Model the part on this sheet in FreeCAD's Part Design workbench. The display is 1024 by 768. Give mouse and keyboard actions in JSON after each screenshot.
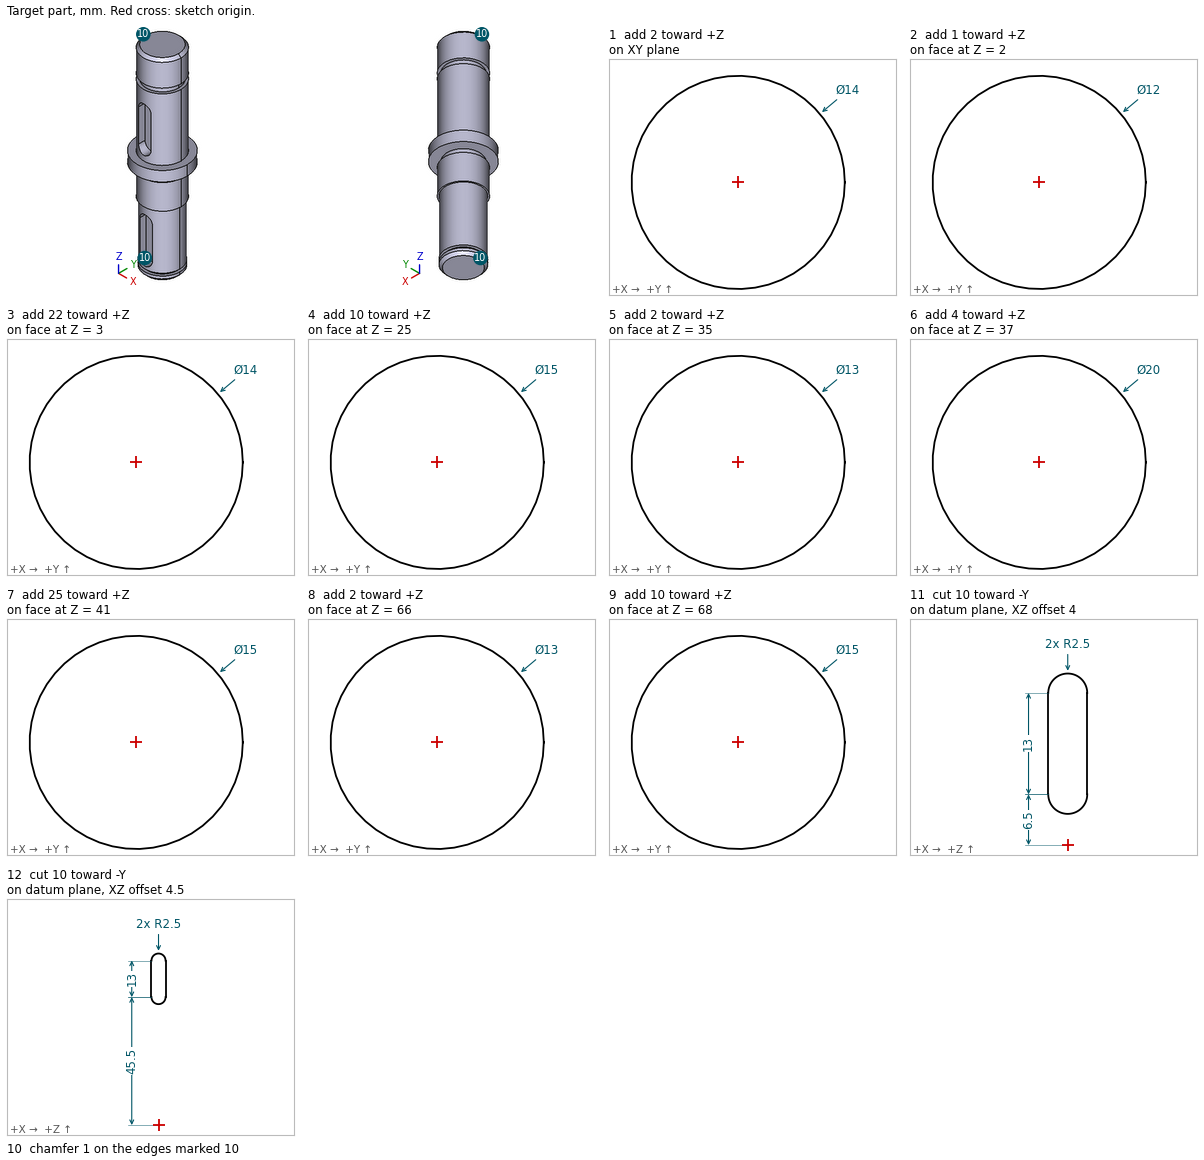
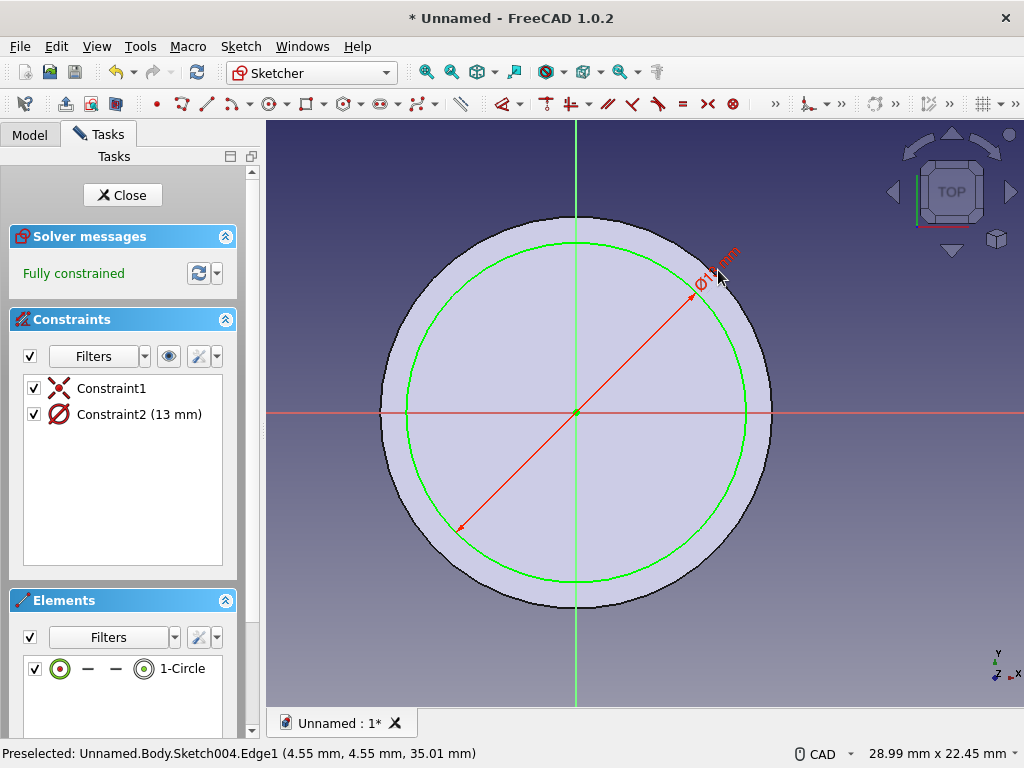
{"action": "left_click", "coordinate": [123, 195]}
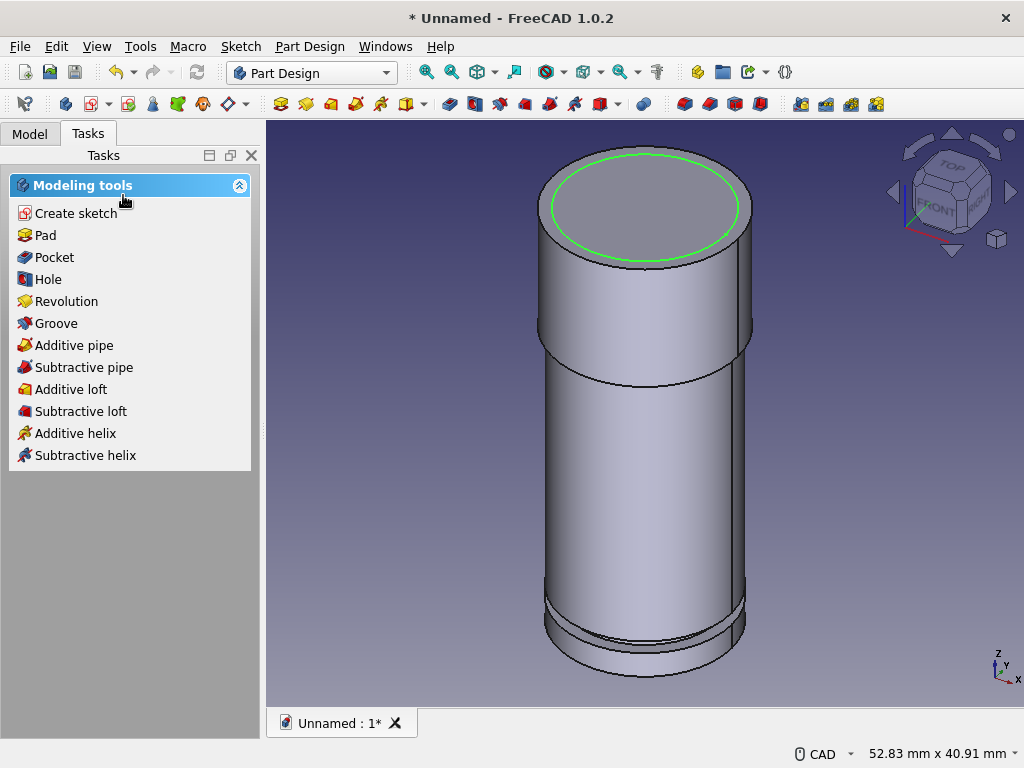
{"action": "left_click", "coordinate": [281, 104]}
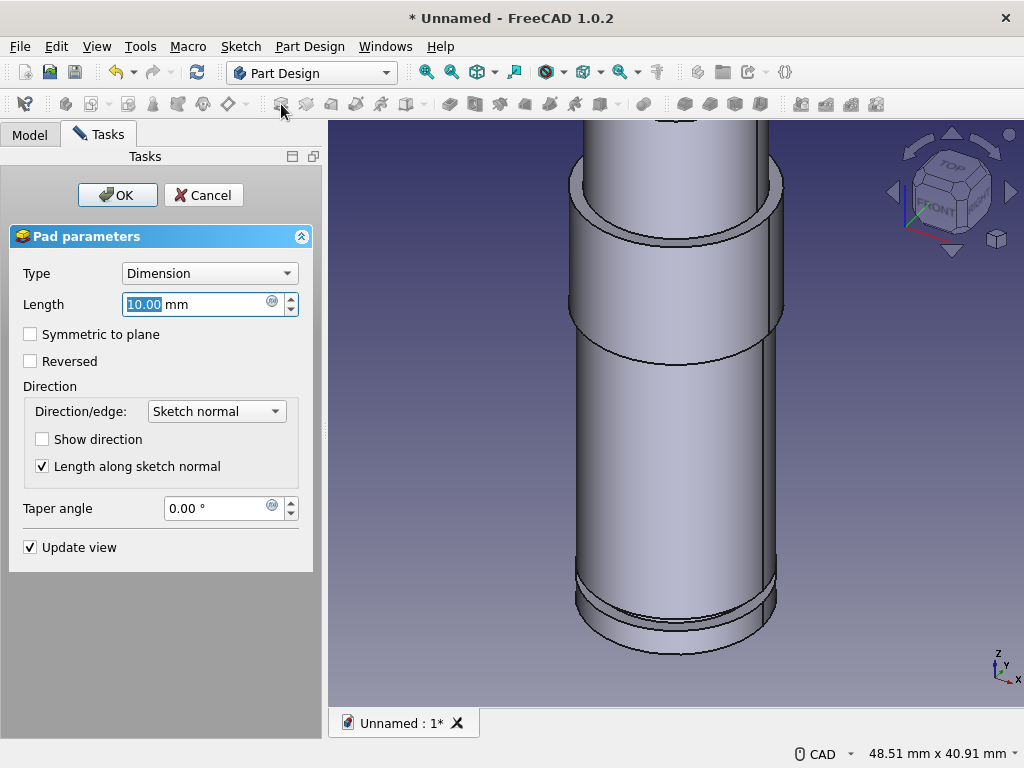
{"action": "type", "text": "2"}
{"action": "key", "text": "Tab"}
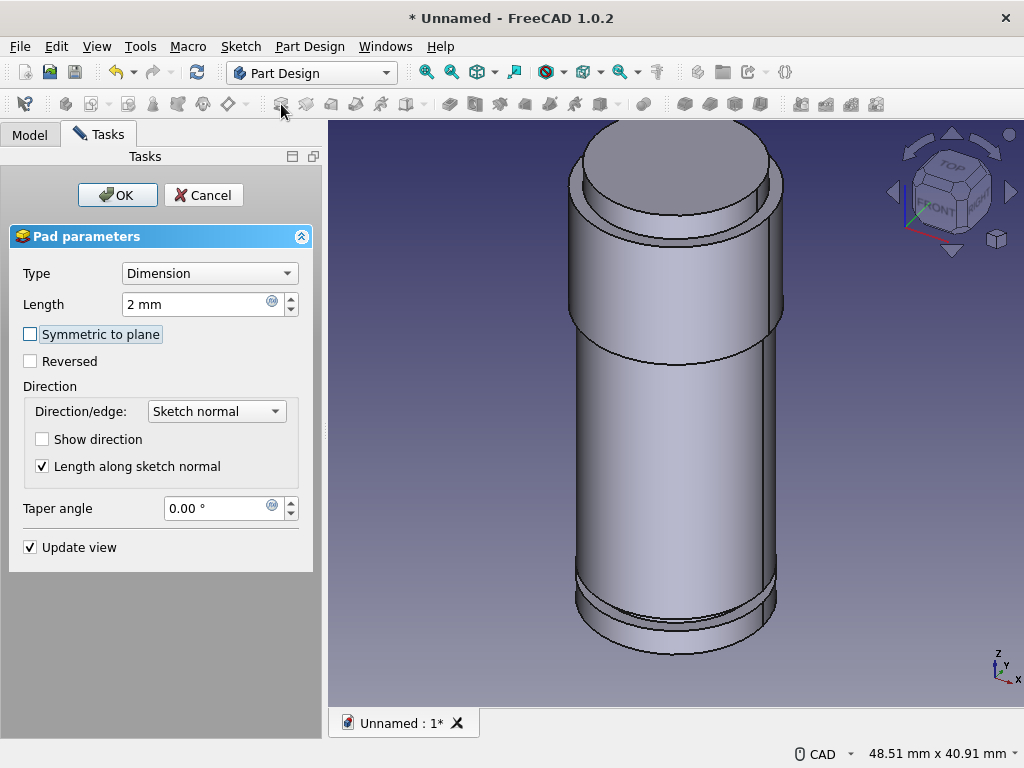
{"action": "left_click", "coordinate": [118, 195]}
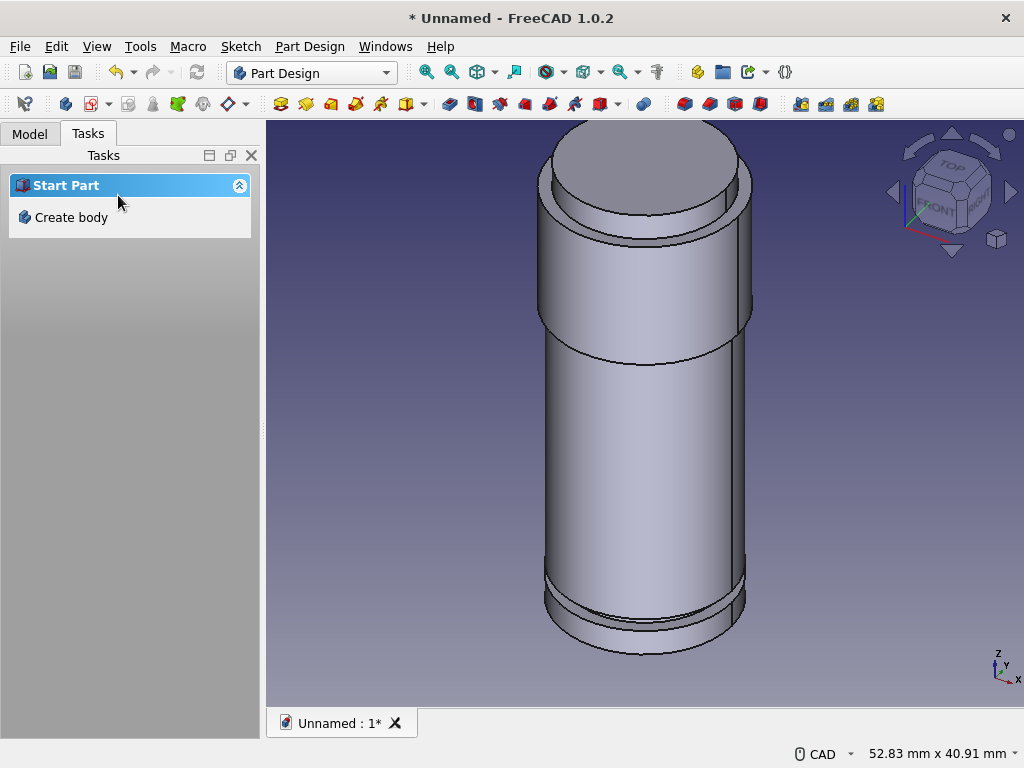
{"action": "left_click", "coordinate": [427, 72]}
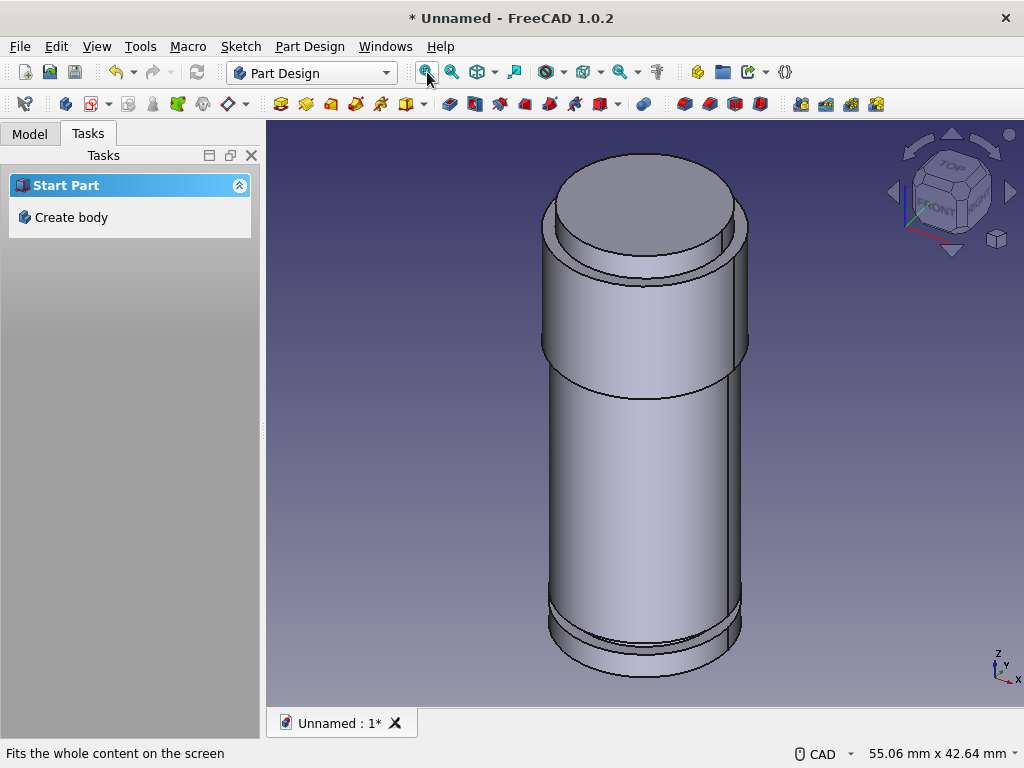
{"action": "left_click", "coordinate": [645, 204]}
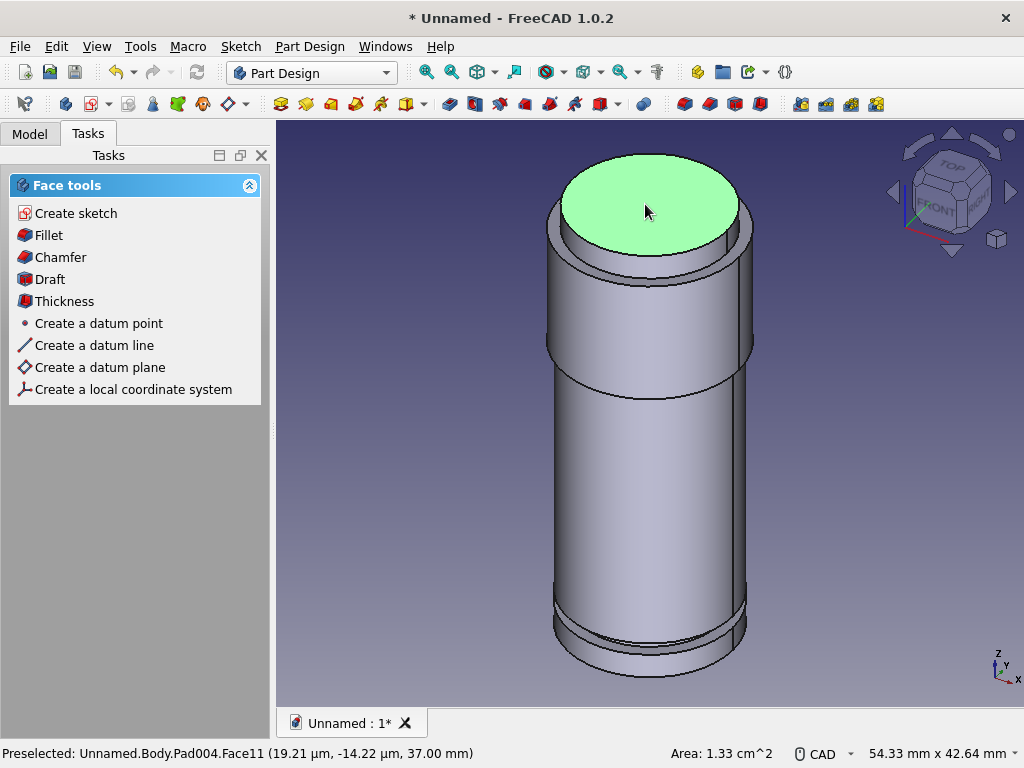
{"action": "left_click", "coordinate": [90, 104]}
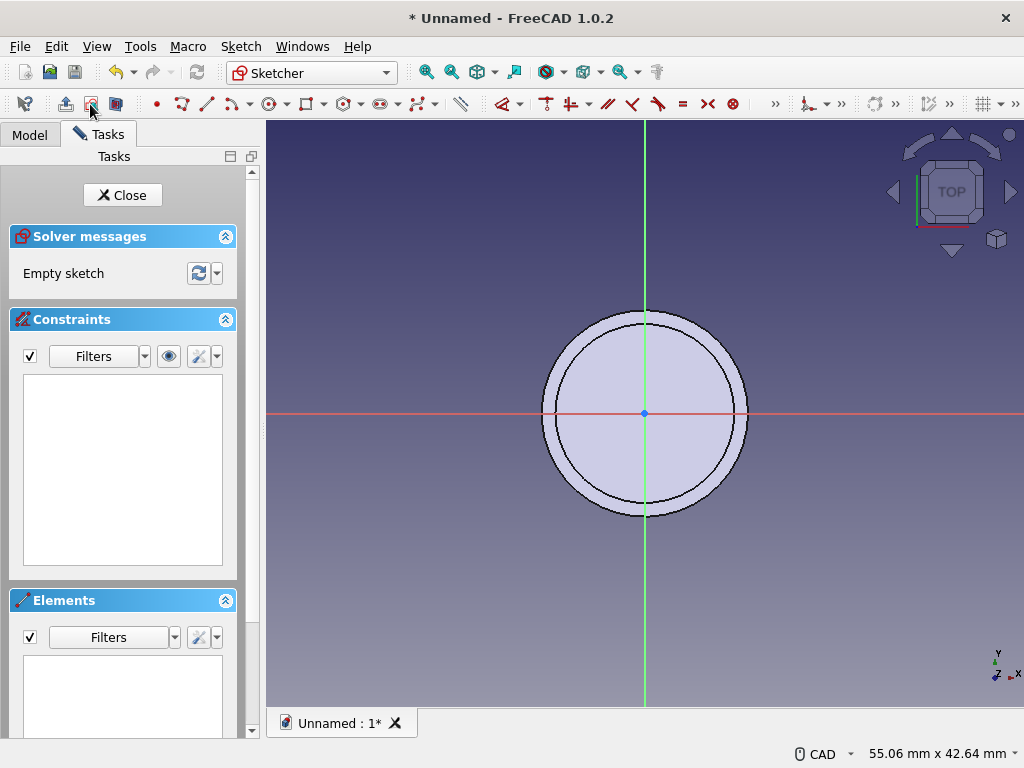
{"action": "scroll", "coordinate": [784, 413], "scroll_direction": "up", "scroll_amount": 2}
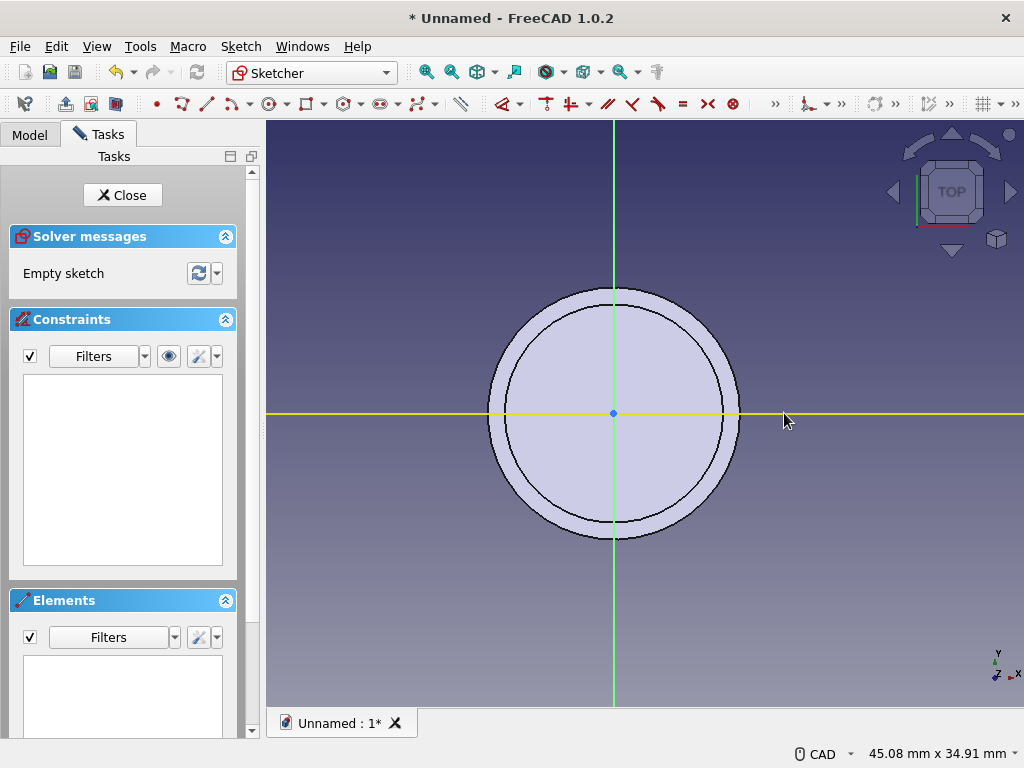
{"action": "left_click", "coordinate": [268, 104]}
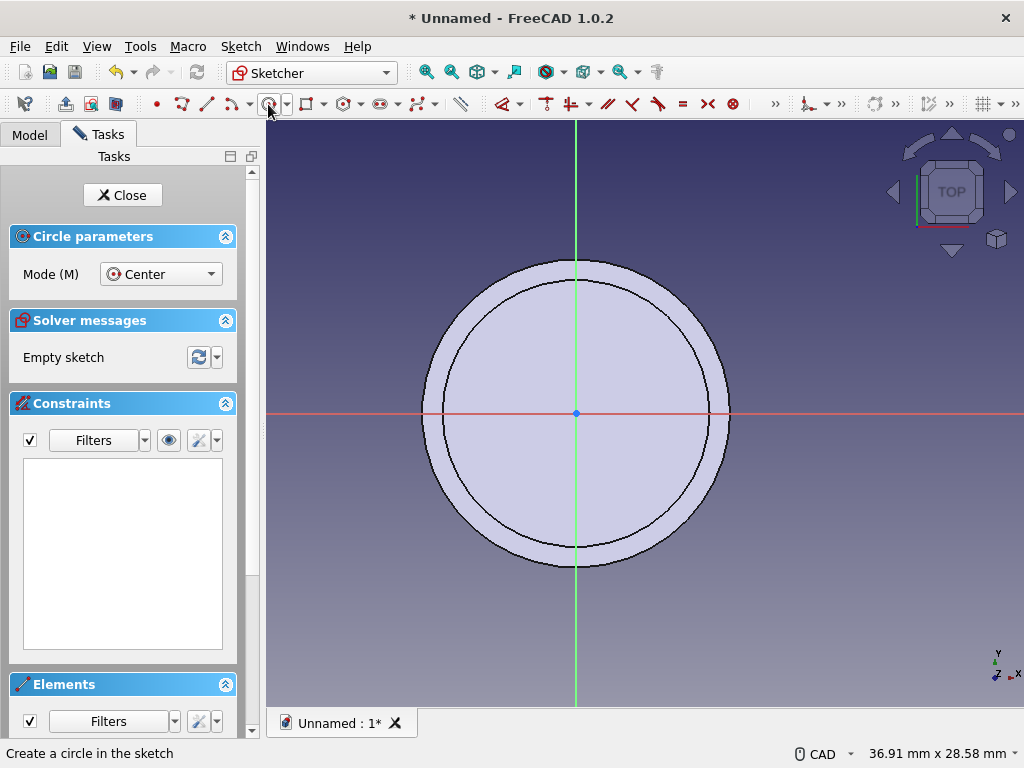
{"action": "left_click", "coordinate": [576, 414]}
{"action": "left_click", "coordinate": [721, 268]}
{"action": "key", "text": "Escape"}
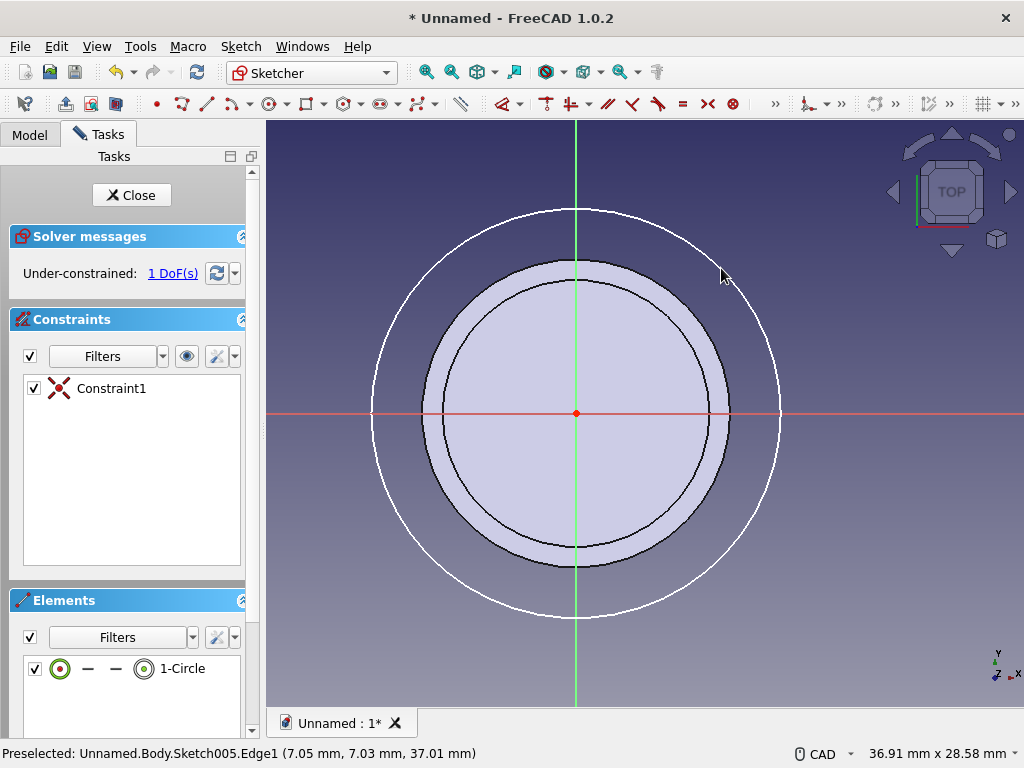
{"action": "left_click", "coordinate": [502, 104]}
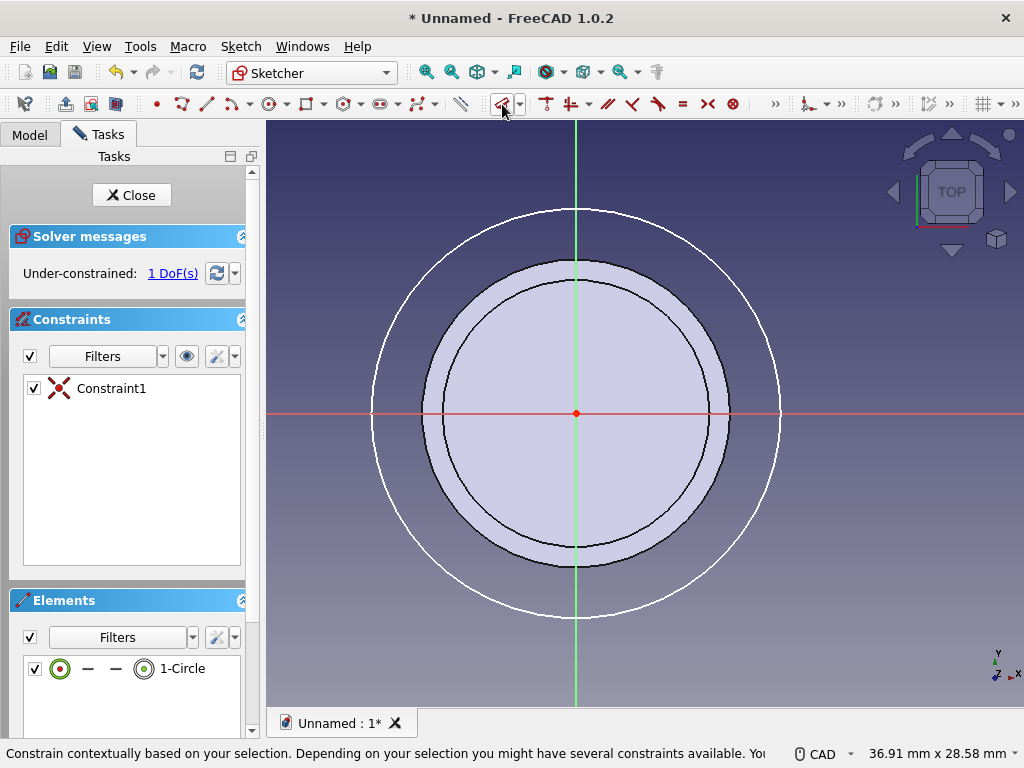
{"action": "left_click", "coordinate": [720, 268]}
{"action": "left_click", "coordinate": [743, 245]}